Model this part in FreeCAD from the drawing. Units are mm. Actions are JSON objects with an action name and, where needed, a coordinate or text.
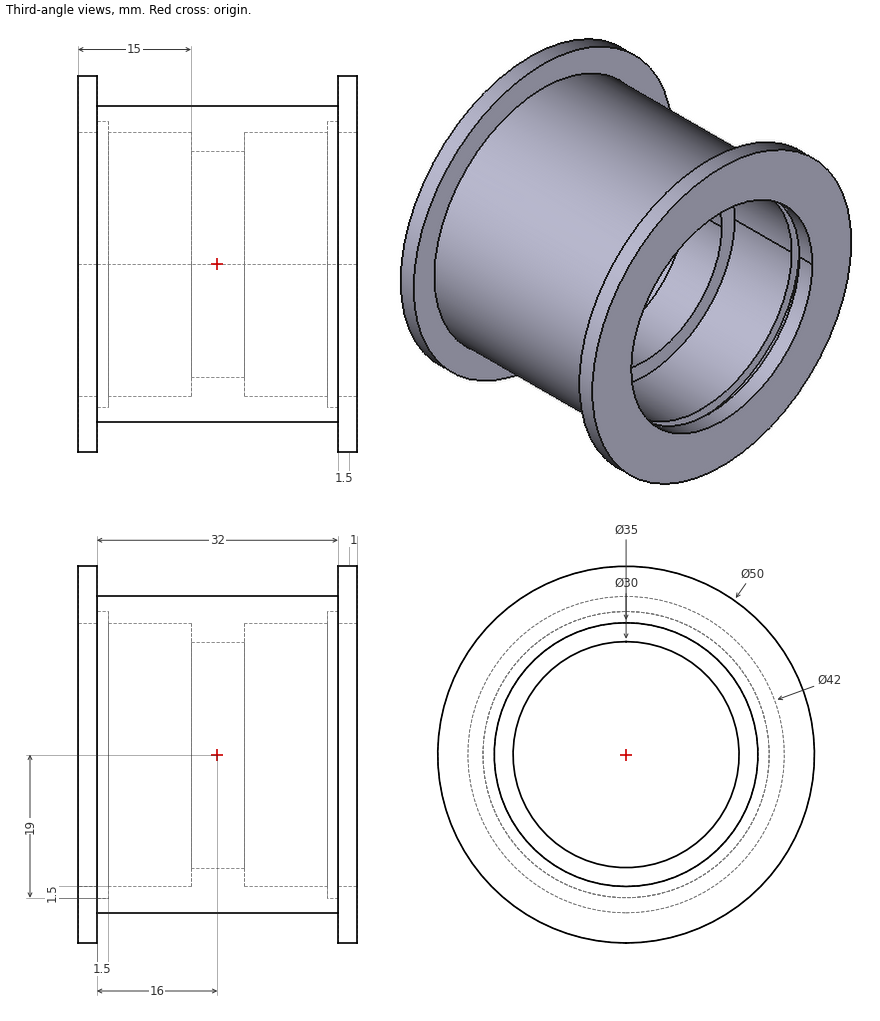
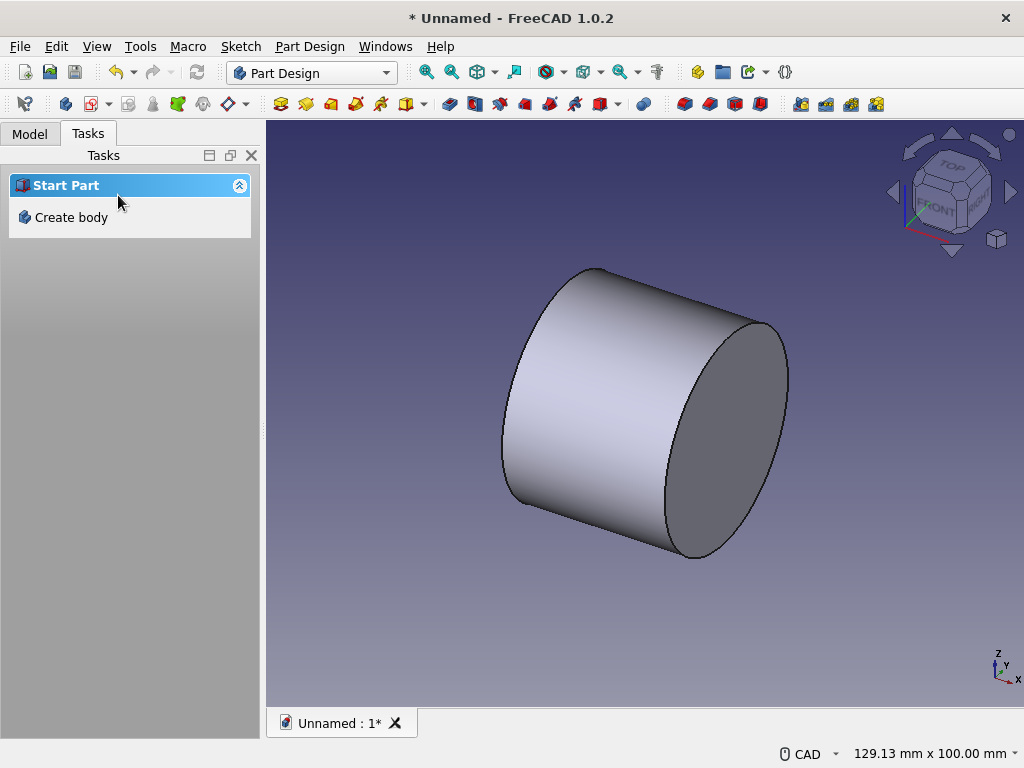
{"action": "left_click", "coordinate": [726, 439]}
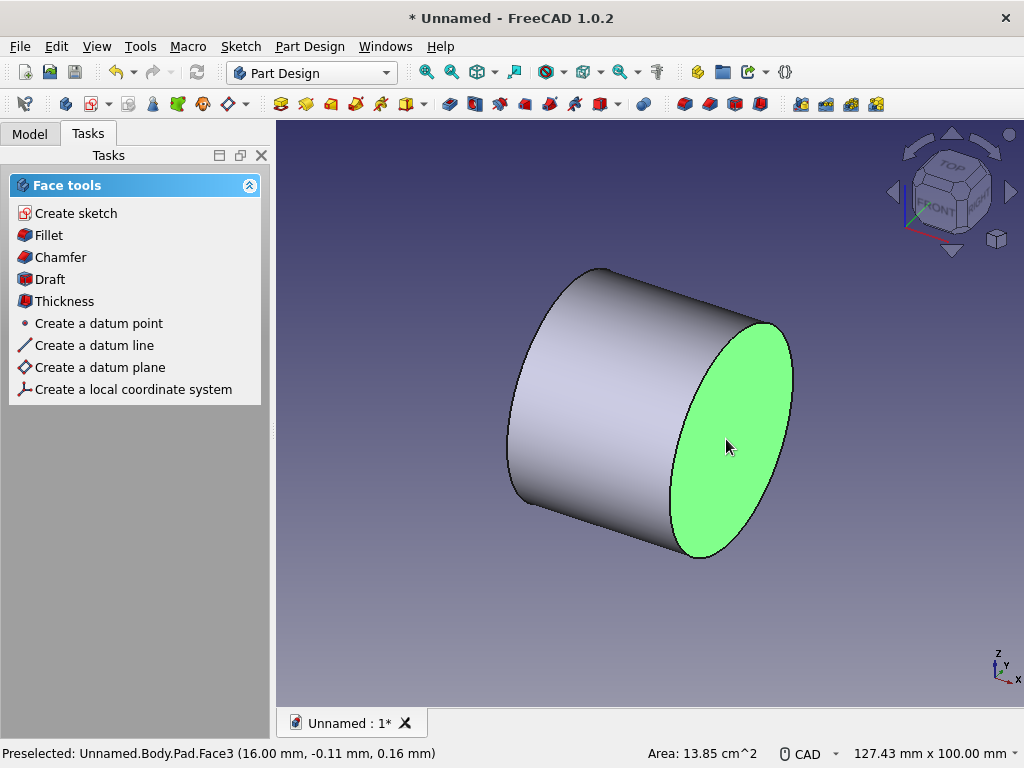
{"action": "left_click", "coordinate": [90, 104]}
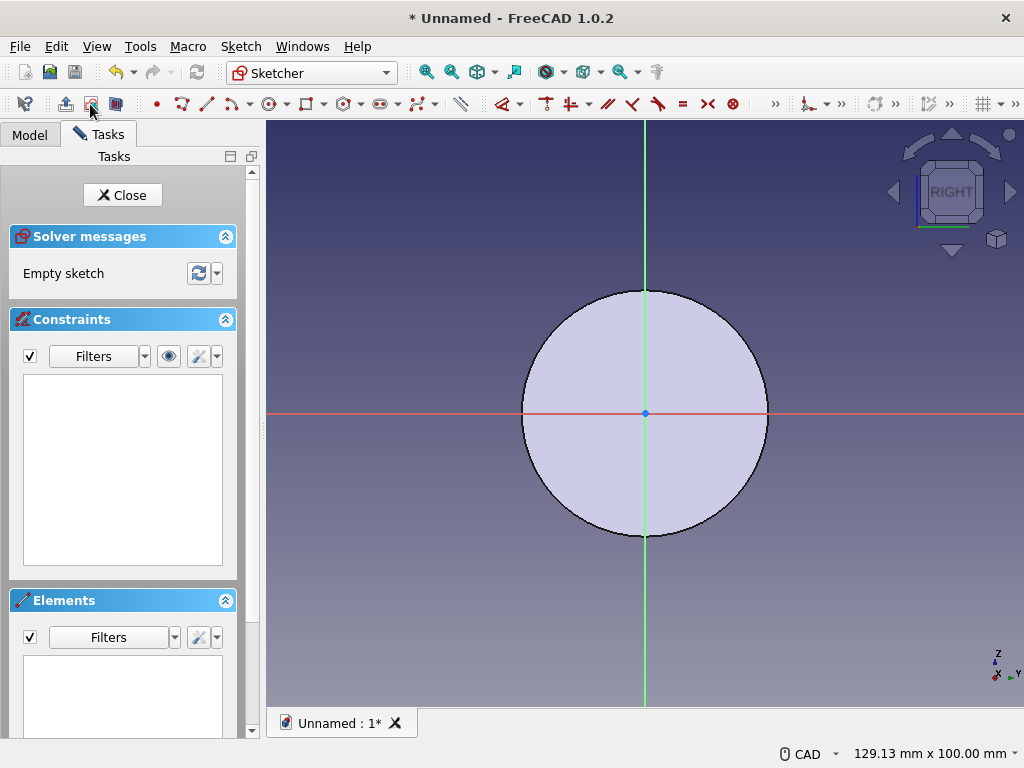
{"action": "left_click", "coordinate": [268, 104]}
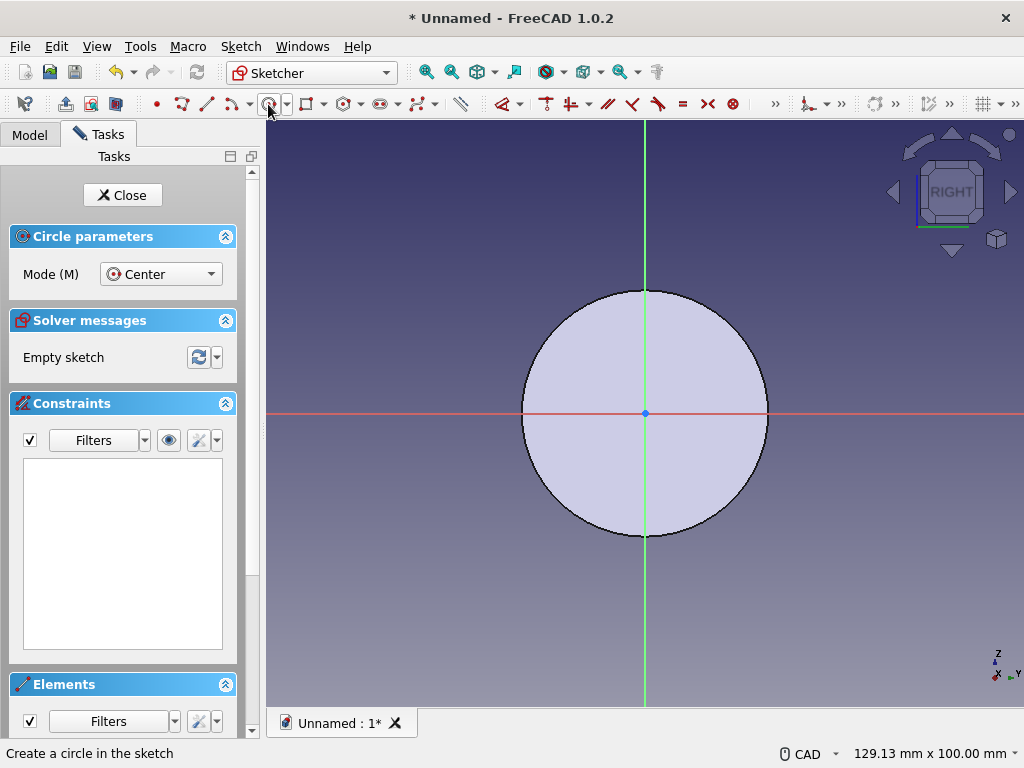
{"action": "left_click", "coordinate": [645, 414]}
{"action": "mouse_move", "coordinate": [749, 310]}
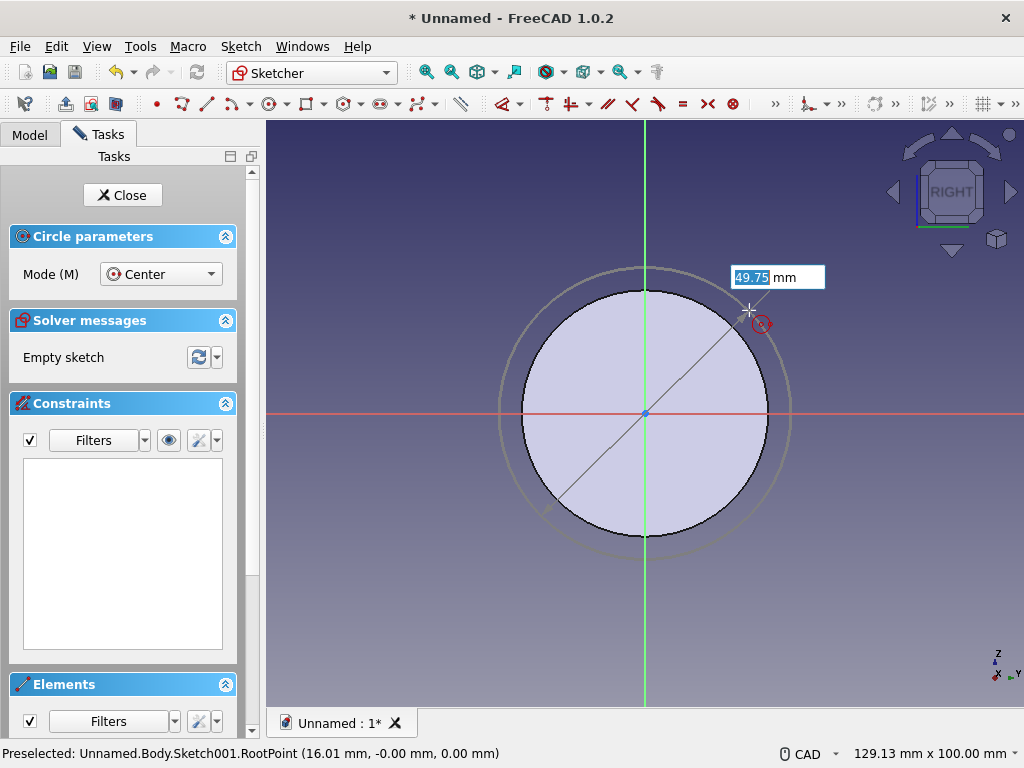
{"action": "type", "text": "50"}
{"action": "key", "text": "Return"}
{"action": "key", "text": "Escape"}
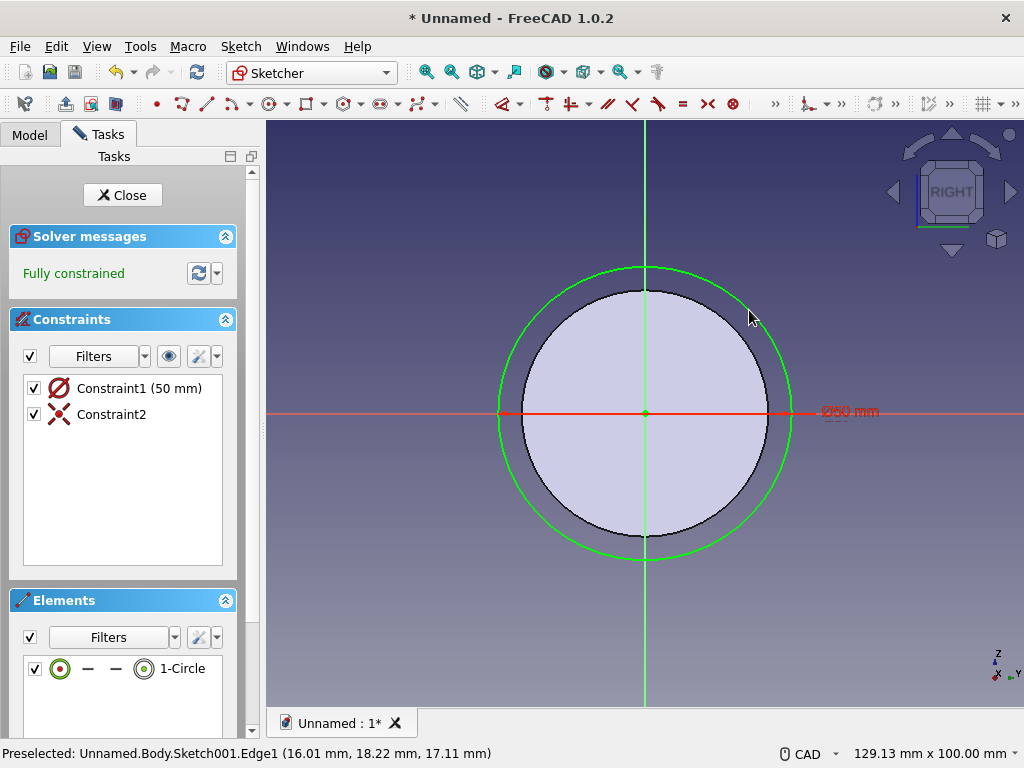
{"action": "left_click", "coordinate": [123, 195]}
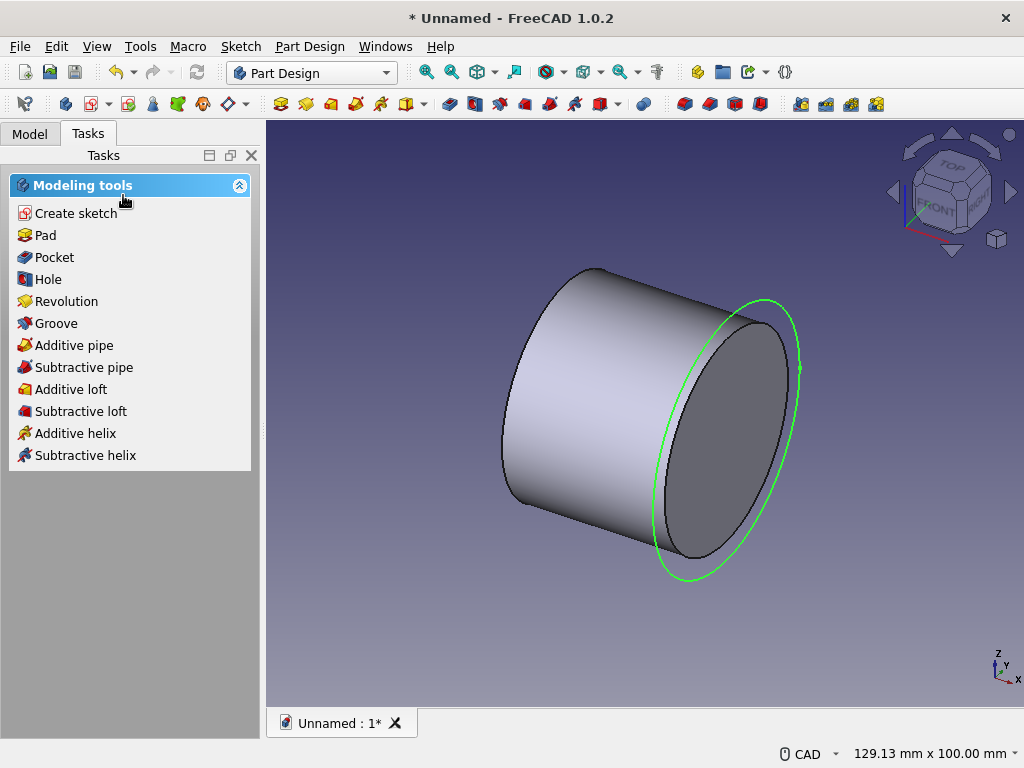
{"action": "left_click", "coordinate": [281, 104]}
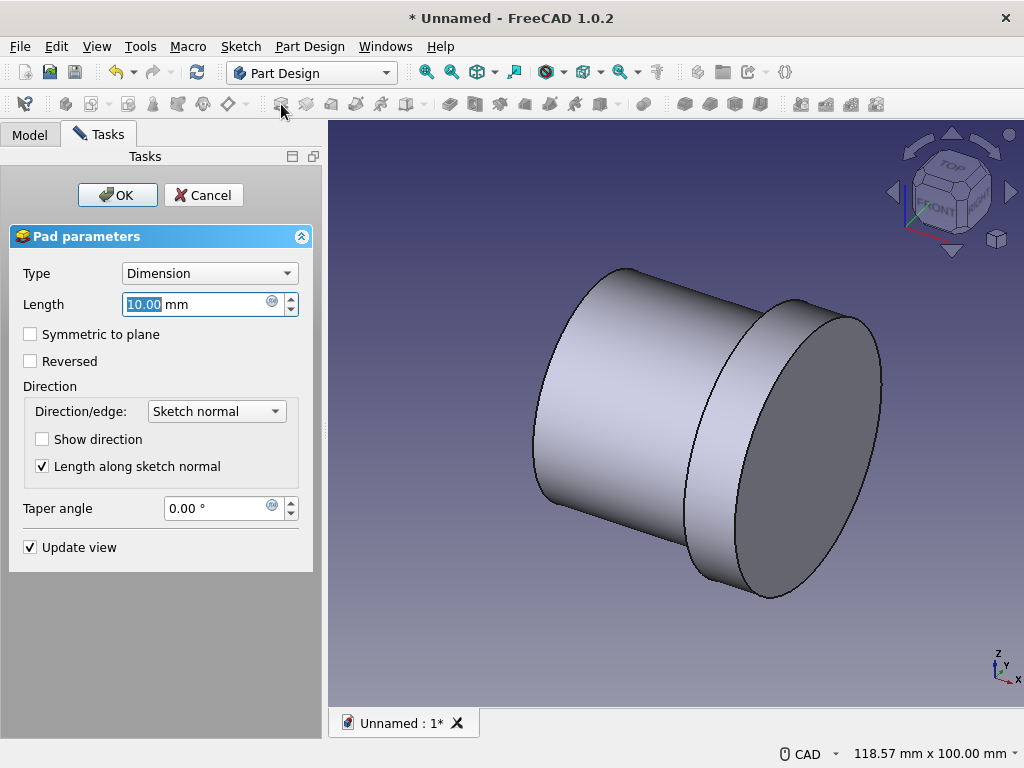
{"action": "type", "text": "1.5"}
{"action": "key", "text": "Tab"}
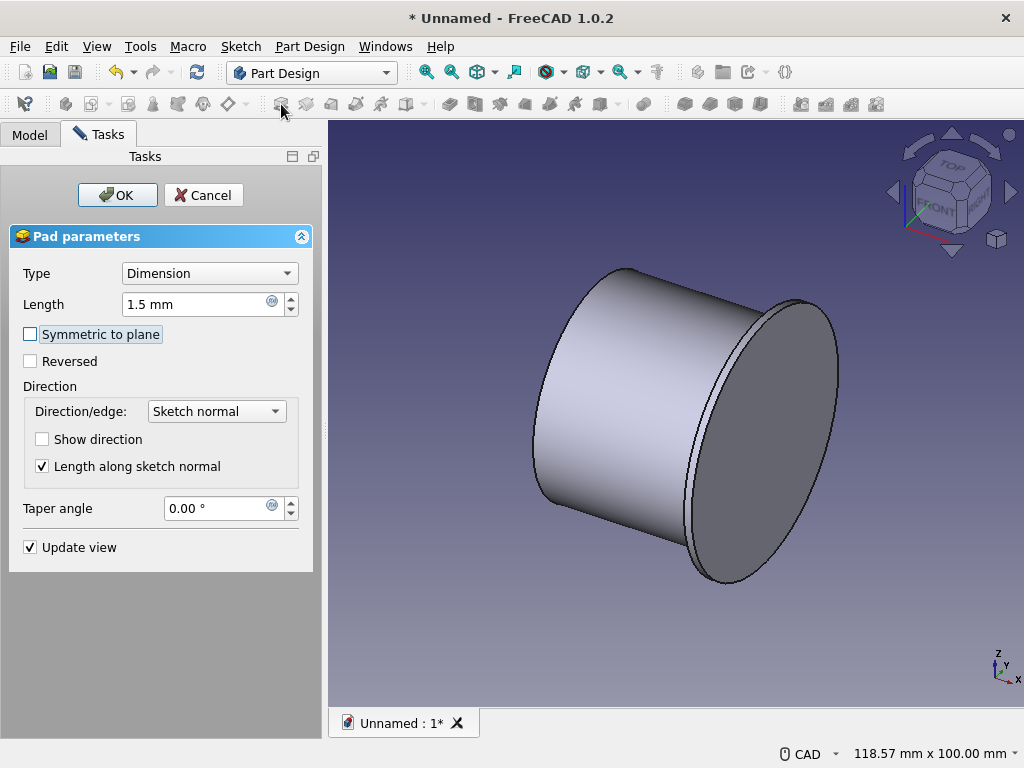
{"action": "left_click", "coordinate": [118, 195]}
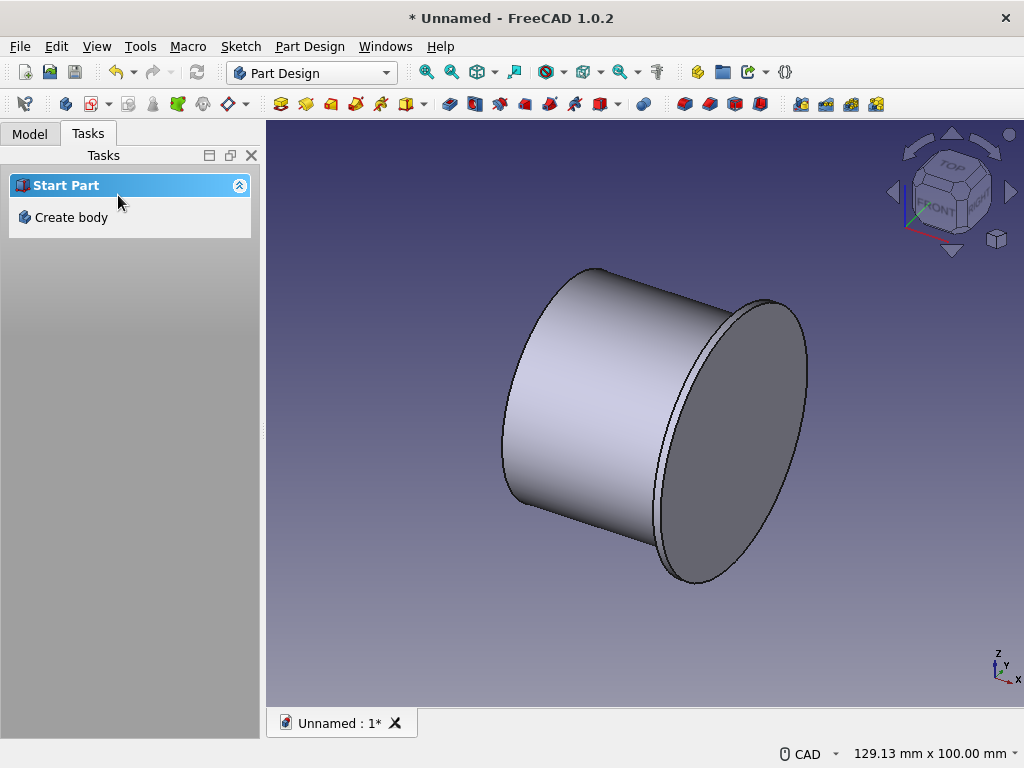
{"action": "left_click", "coordinate": [734, 442]}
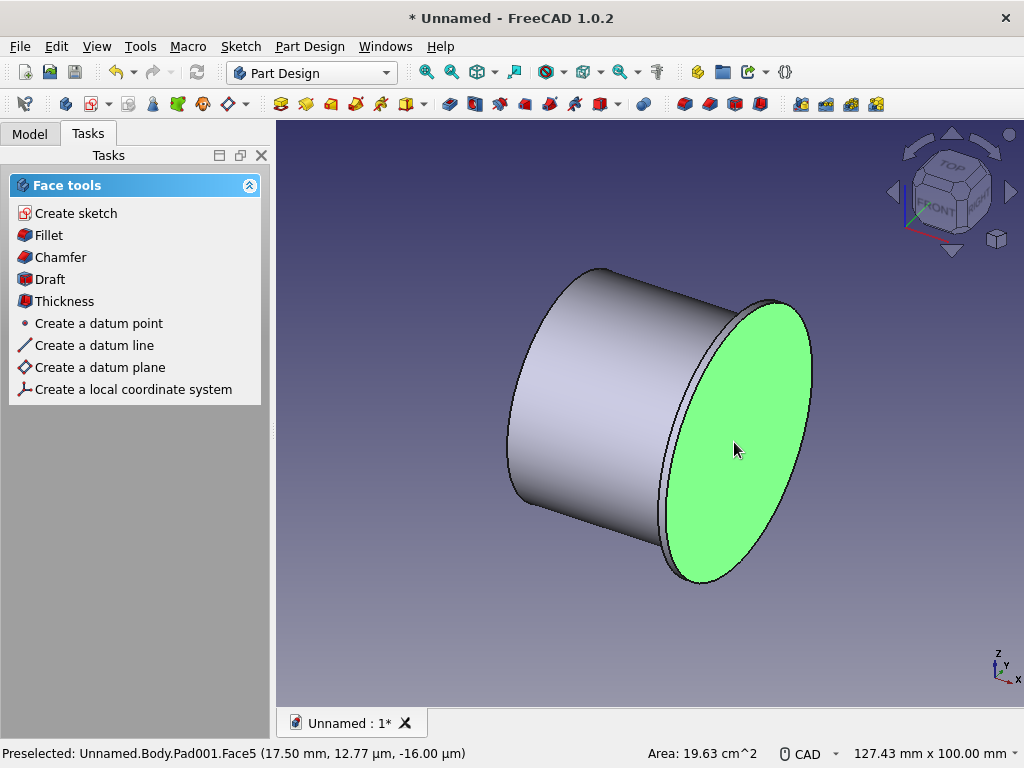
{"action": "left_click", "coordinate": [90, 104]}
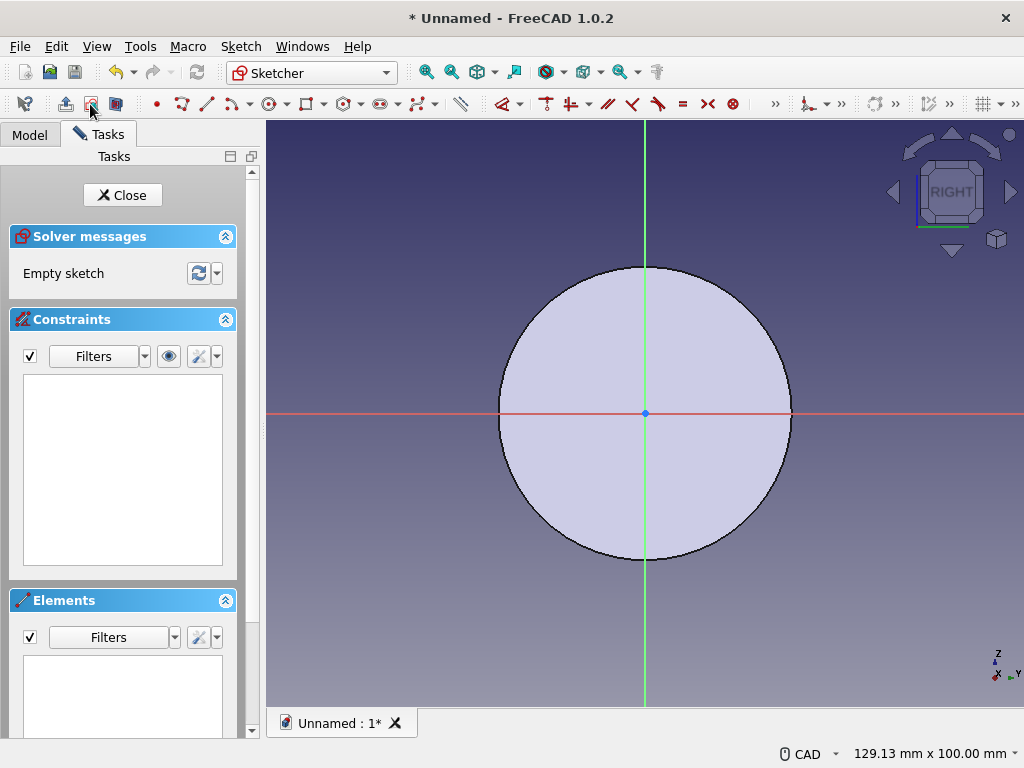
{"action": "key", "text": "g c"}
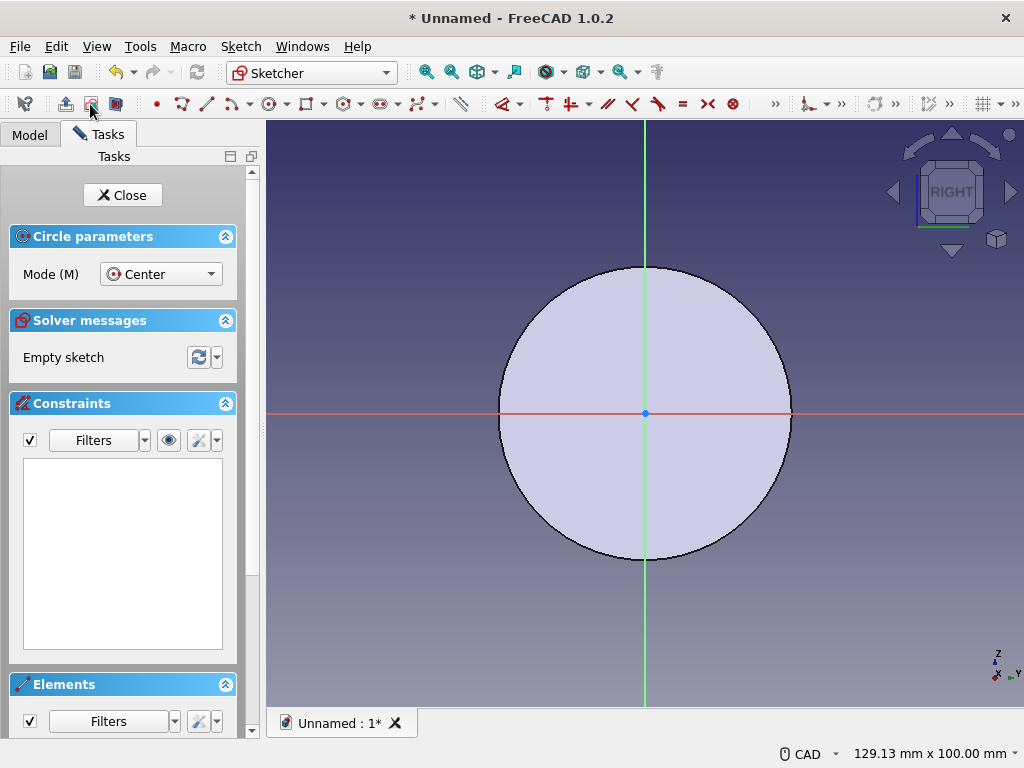
{"action": "left_click", "coordinate": [645, 414]}
{"action": "mouse_move", "coordinate": [749, 310]}